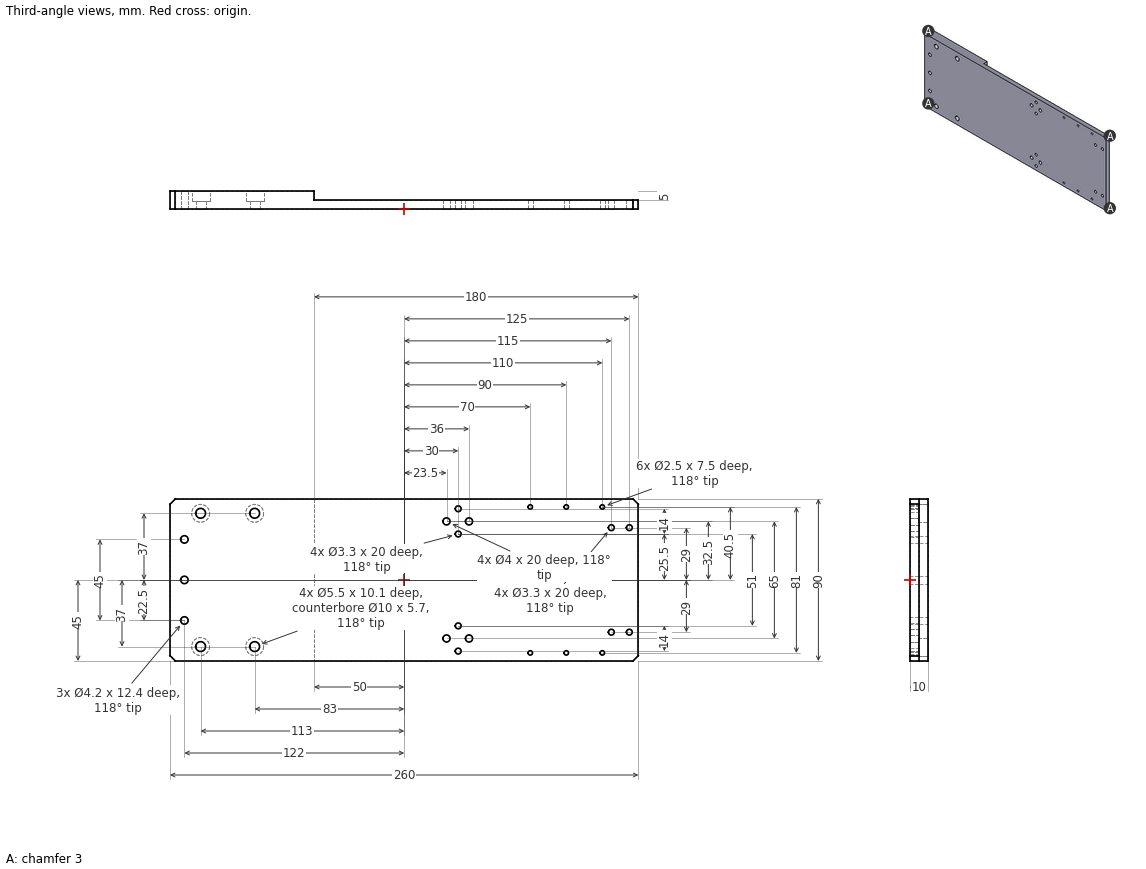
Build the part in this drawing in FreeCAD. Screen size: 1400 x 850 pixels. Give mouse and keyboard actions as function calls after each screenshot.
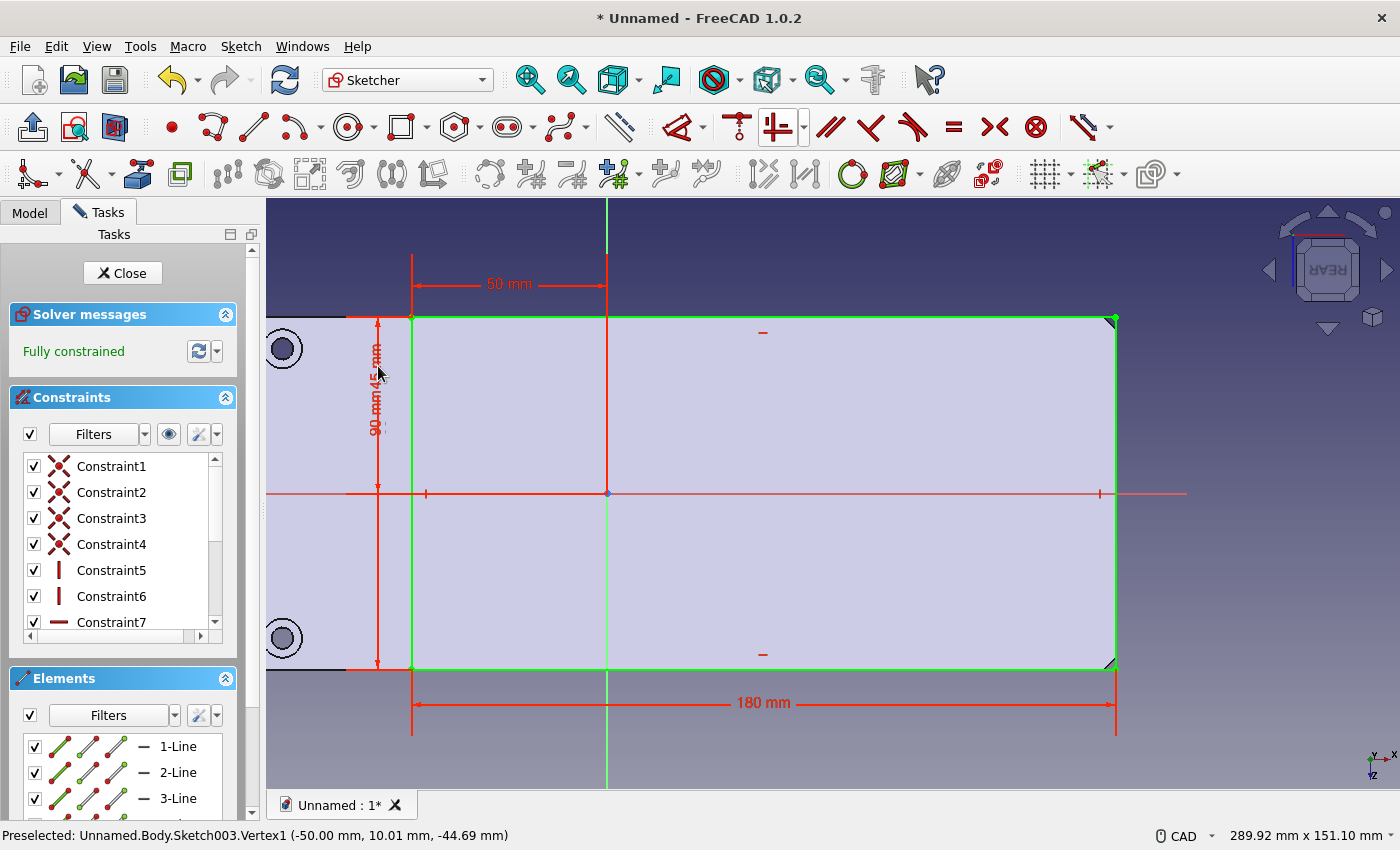
click(123, 273)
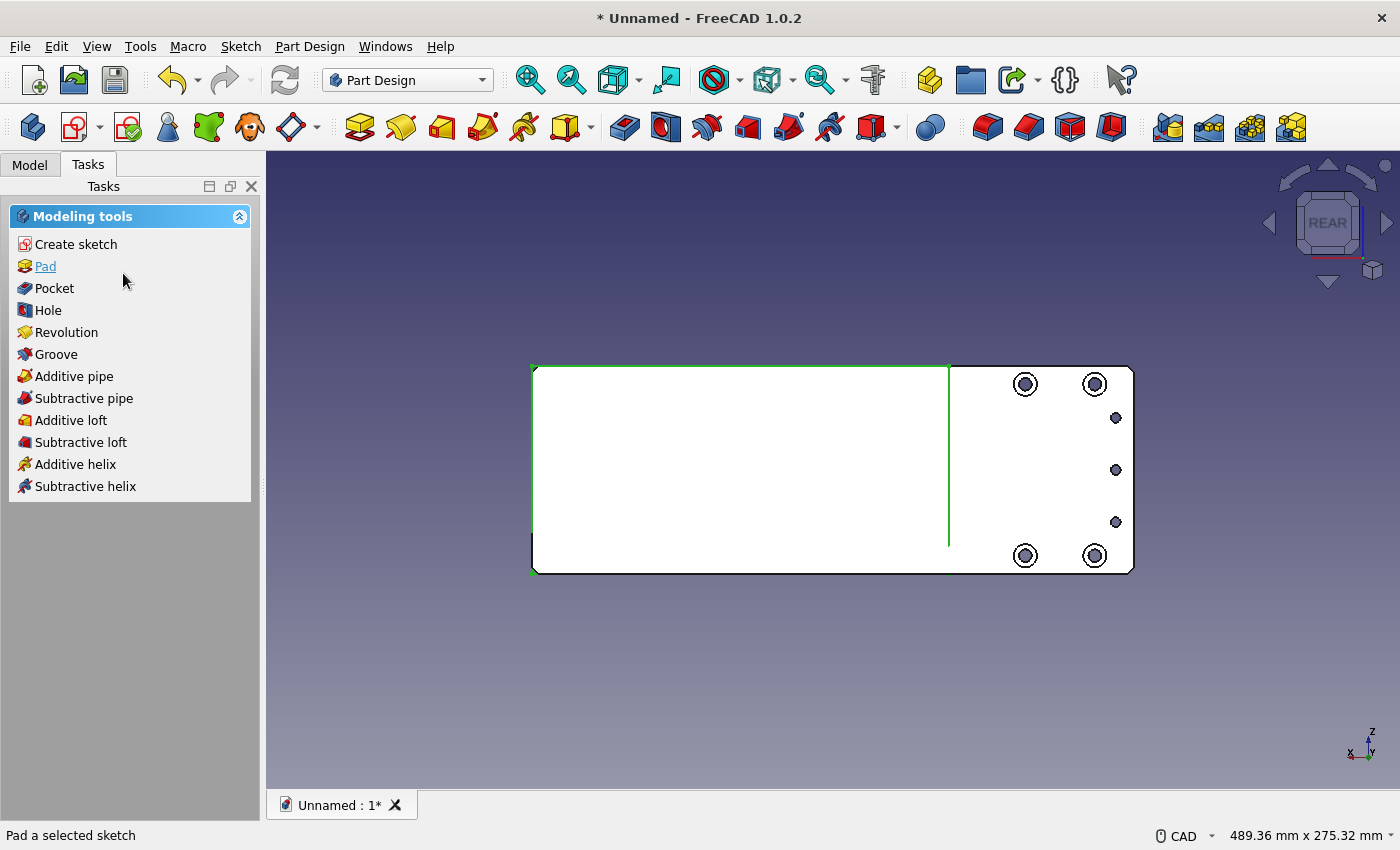
click(625, 128)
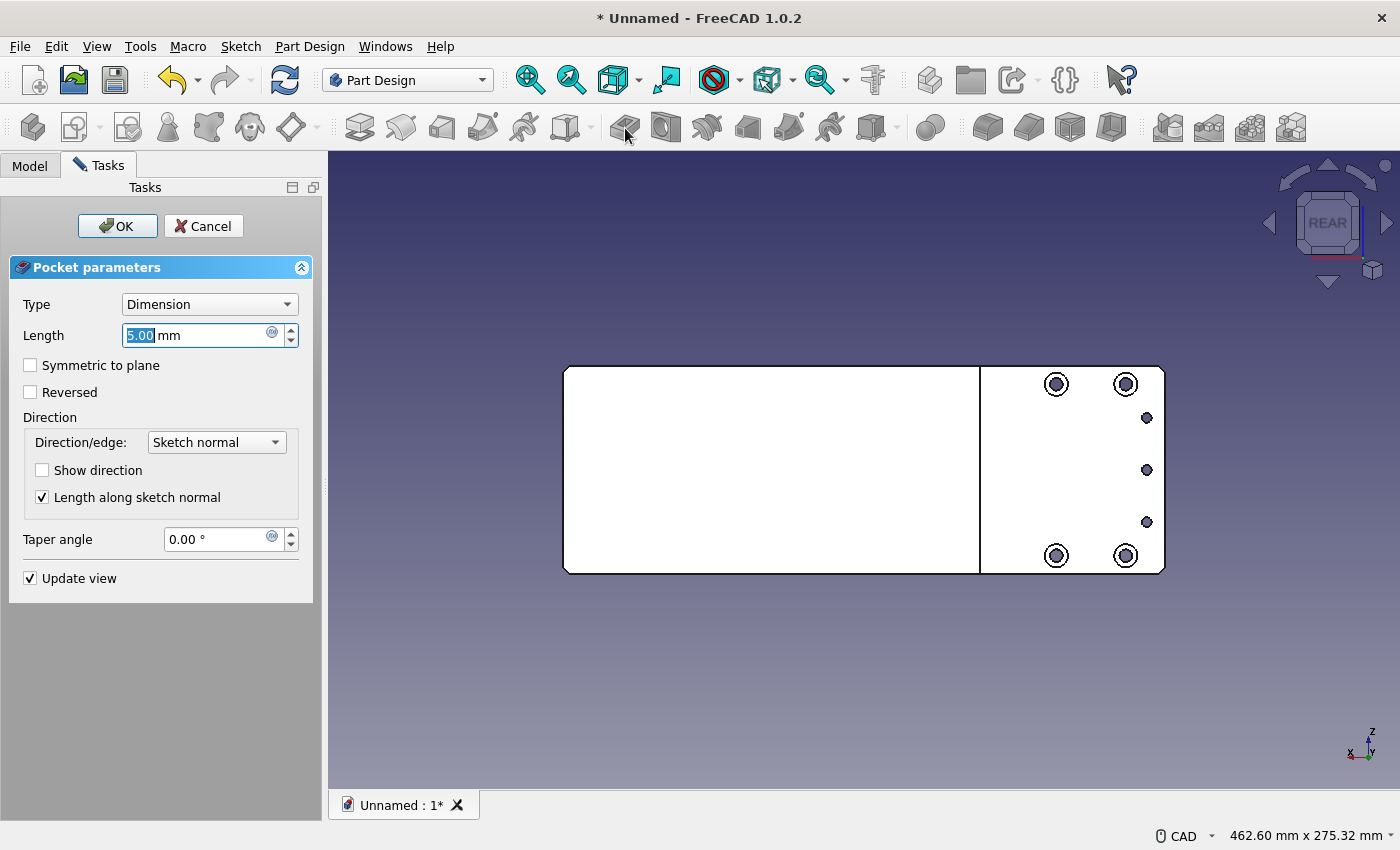
text(5)
key(Tab)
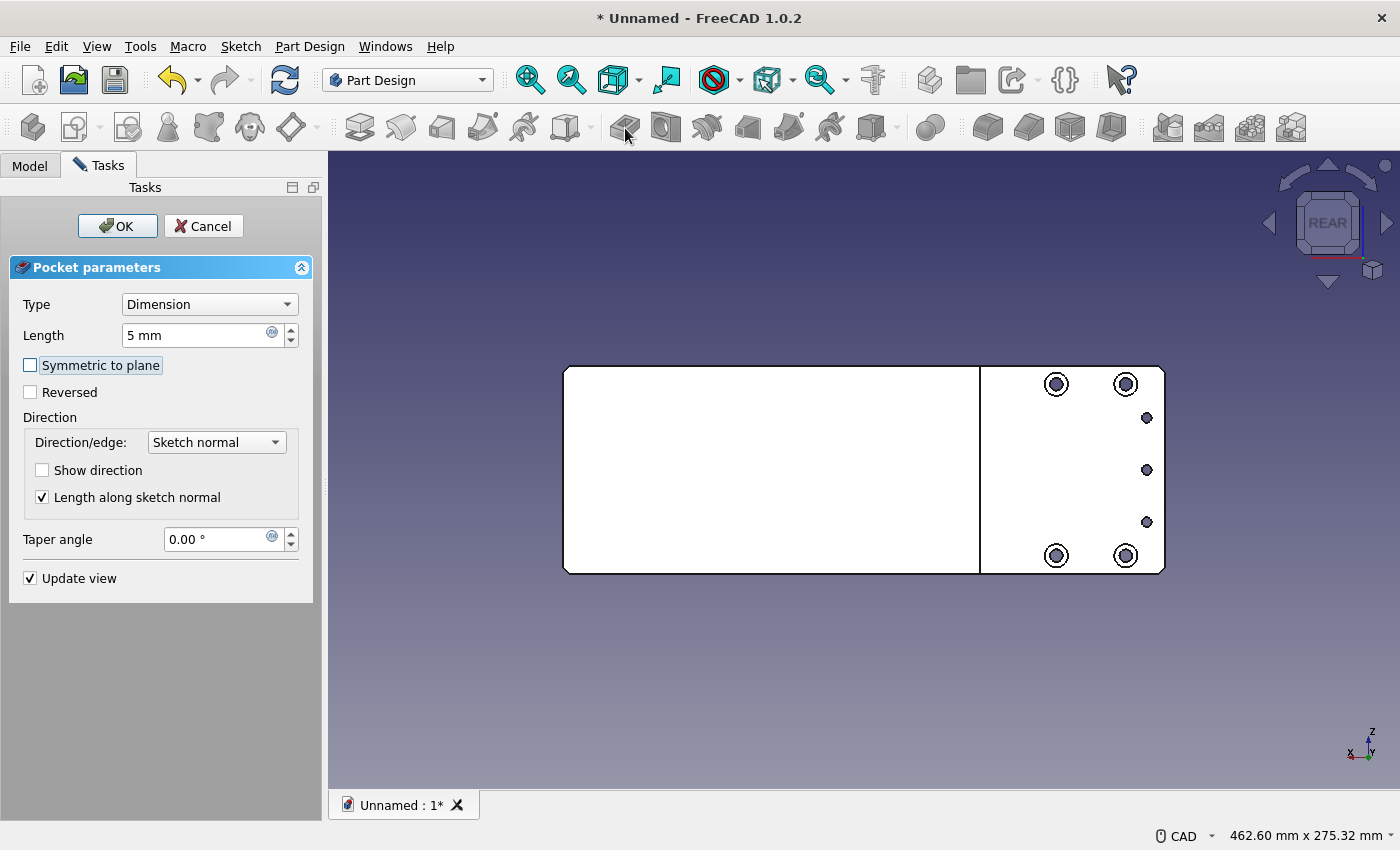
click(118, 226)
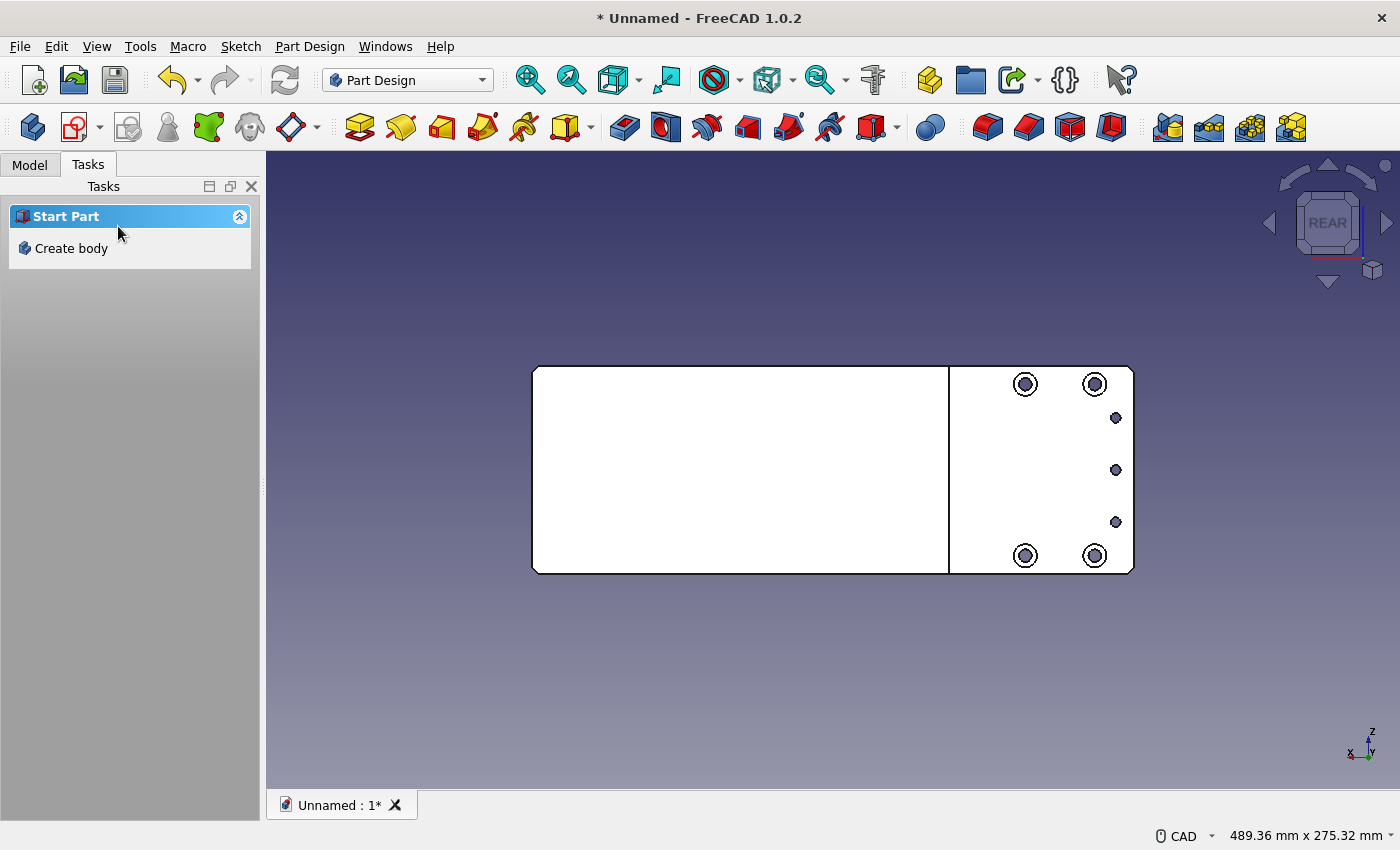
click(681, 469)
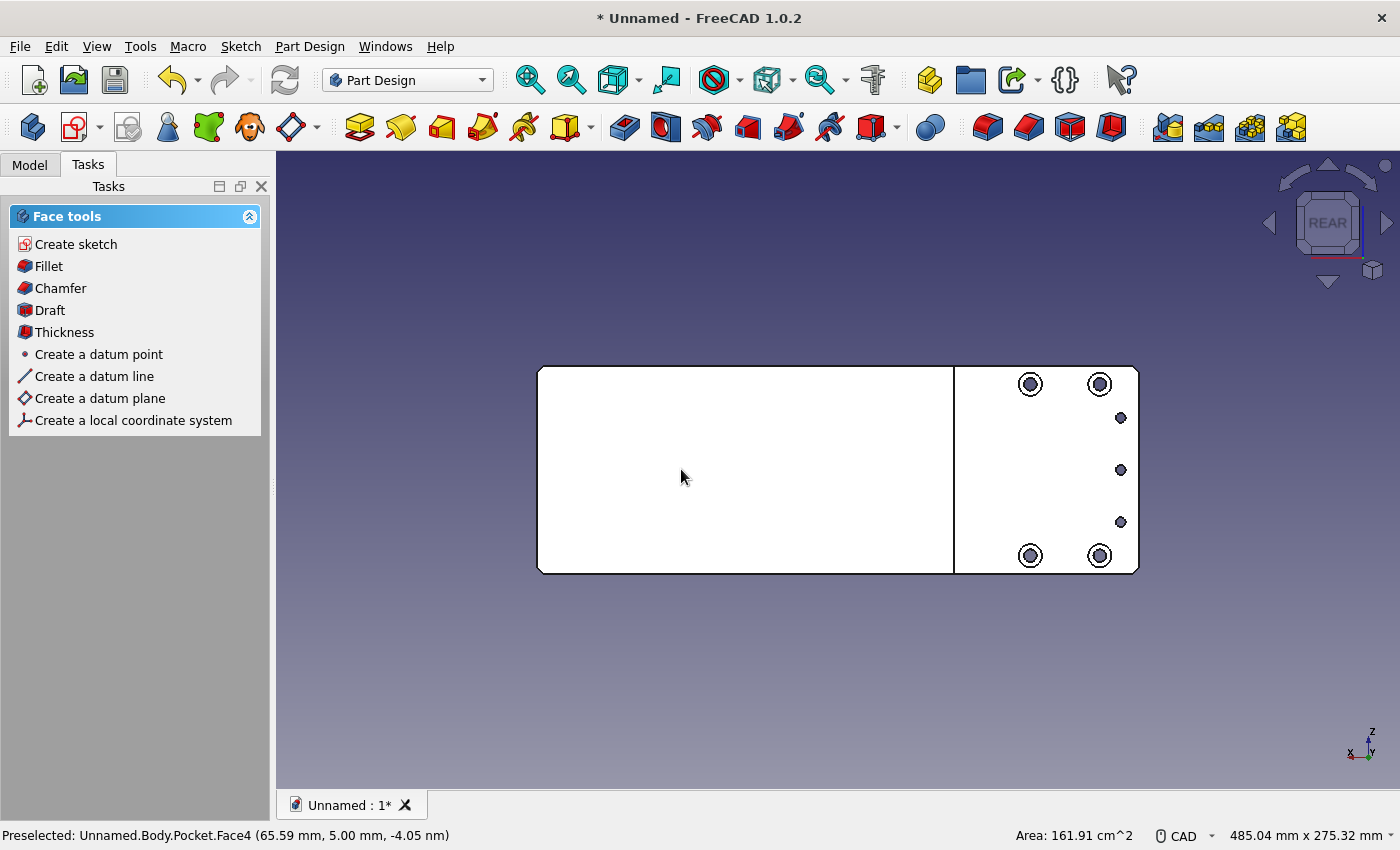
click(74, 128)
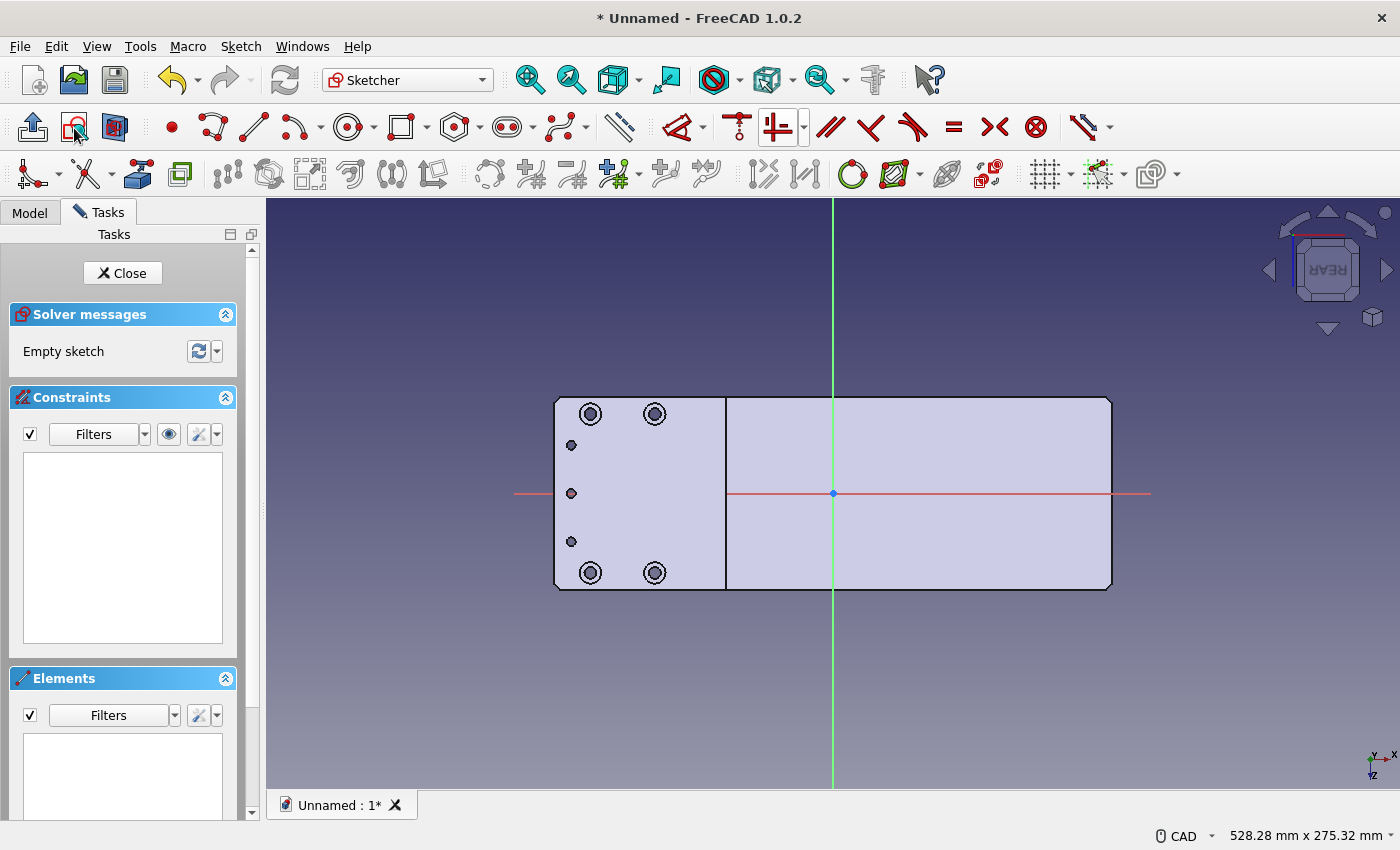
scroll(1106, 493, up, 4)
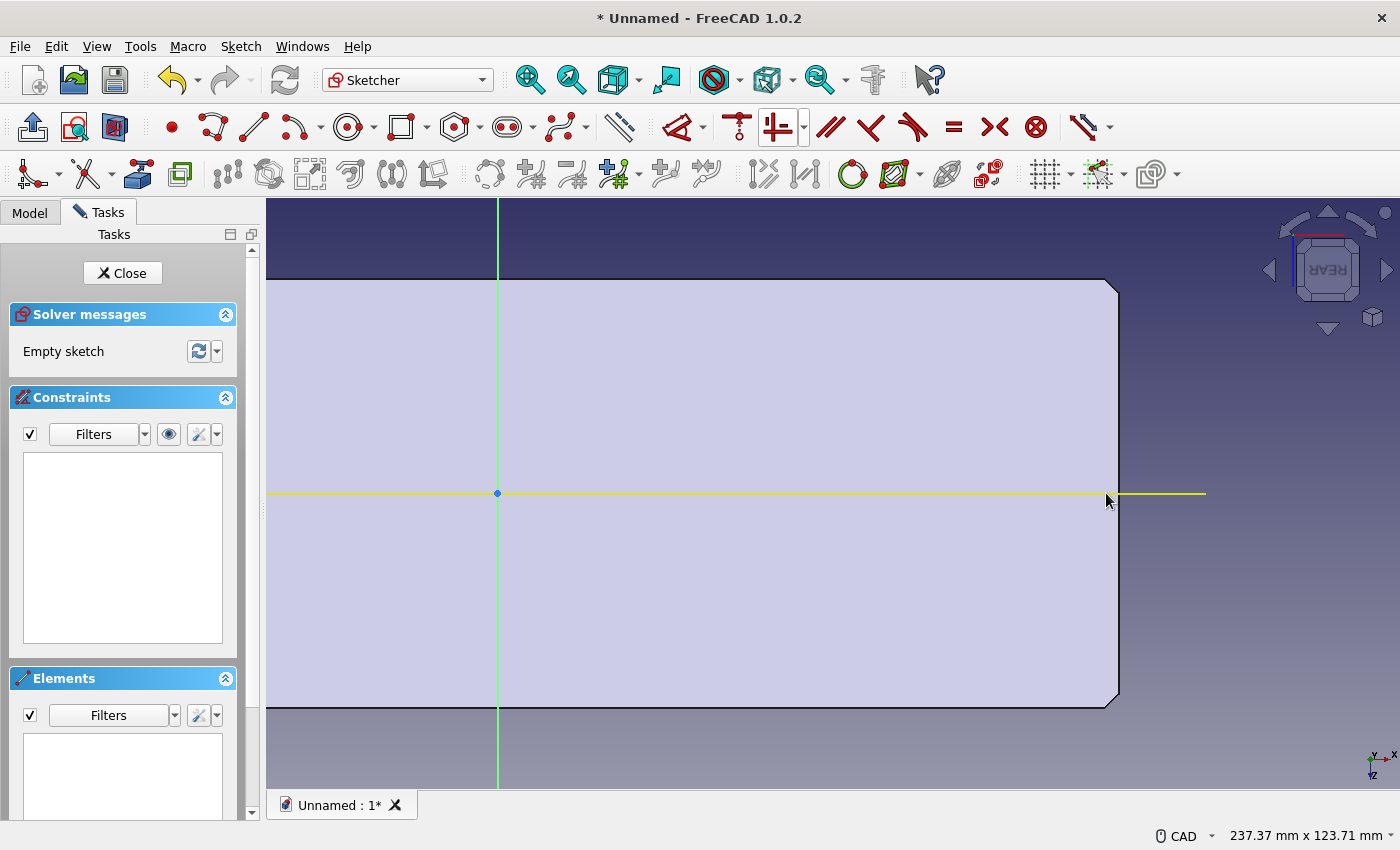
click(348, 128)